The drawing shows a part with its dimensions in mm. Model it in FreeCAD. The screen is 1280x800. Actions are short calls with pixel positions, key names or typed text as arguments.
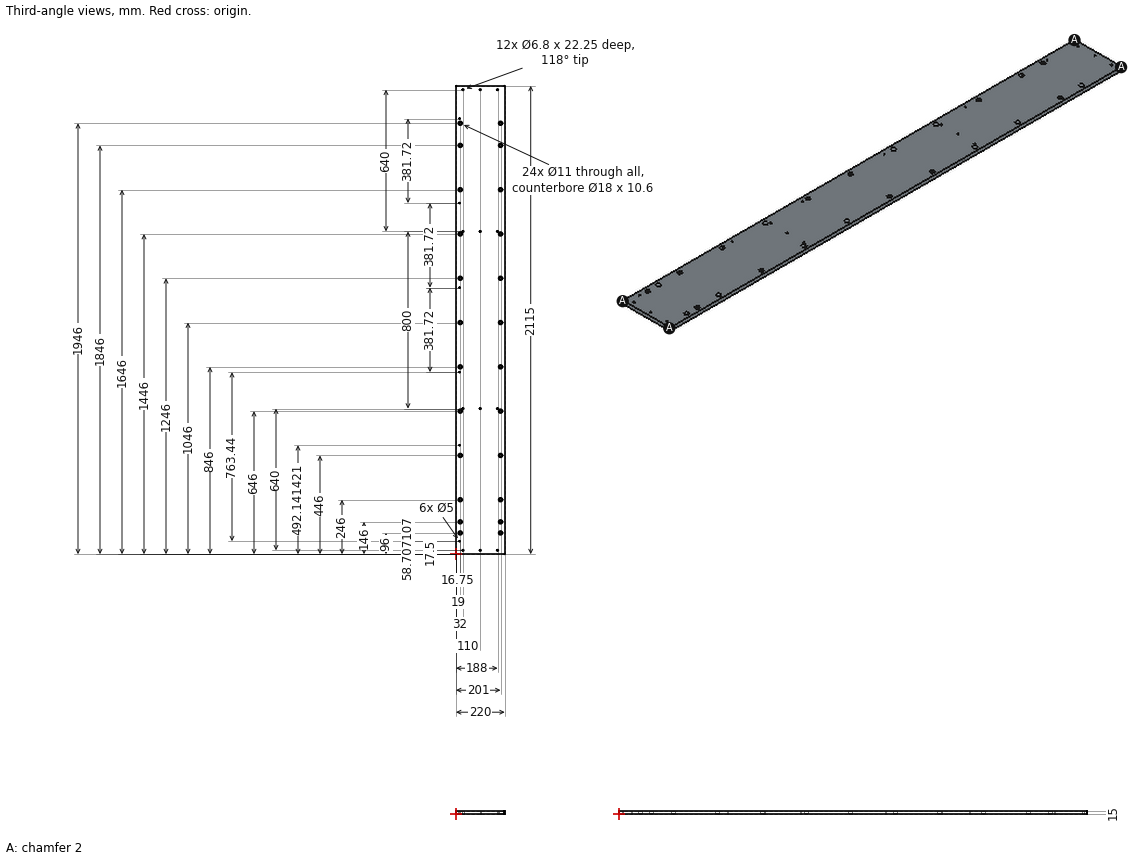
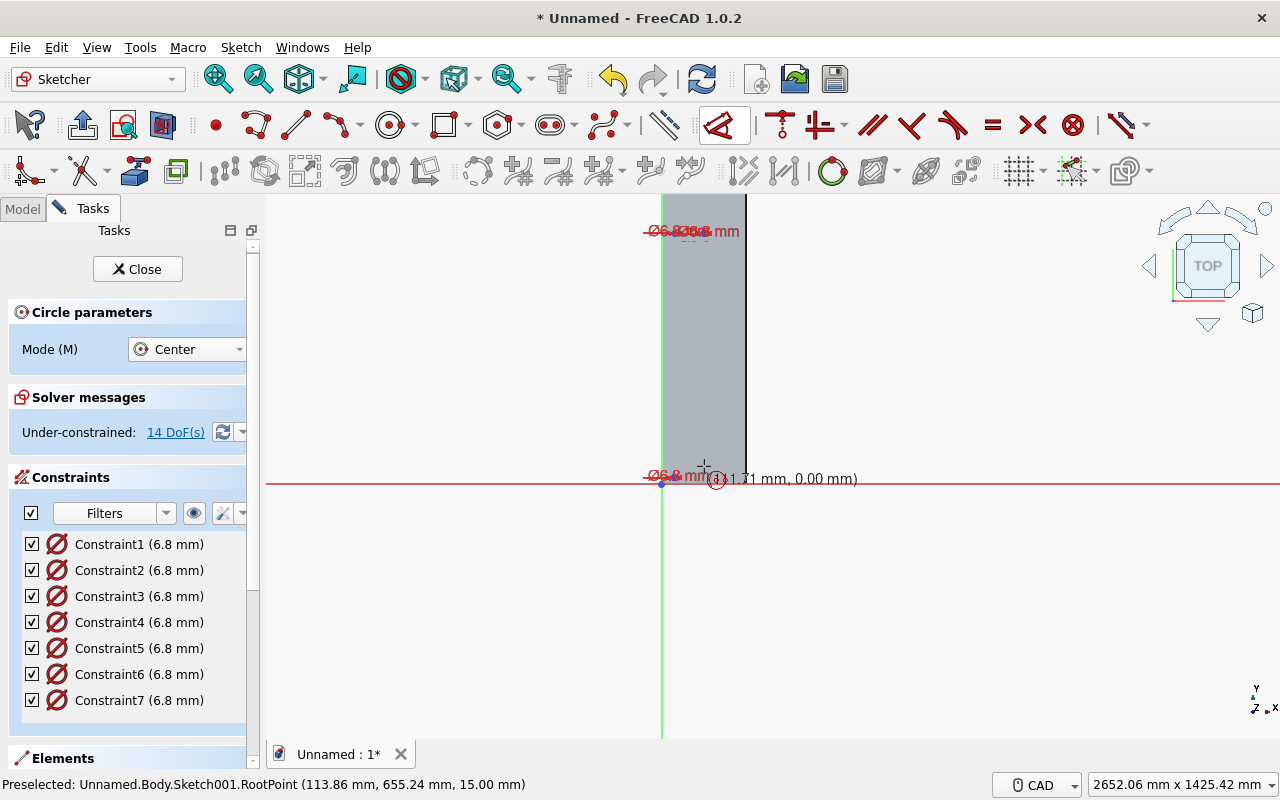
scroll(710, 711, down, 4)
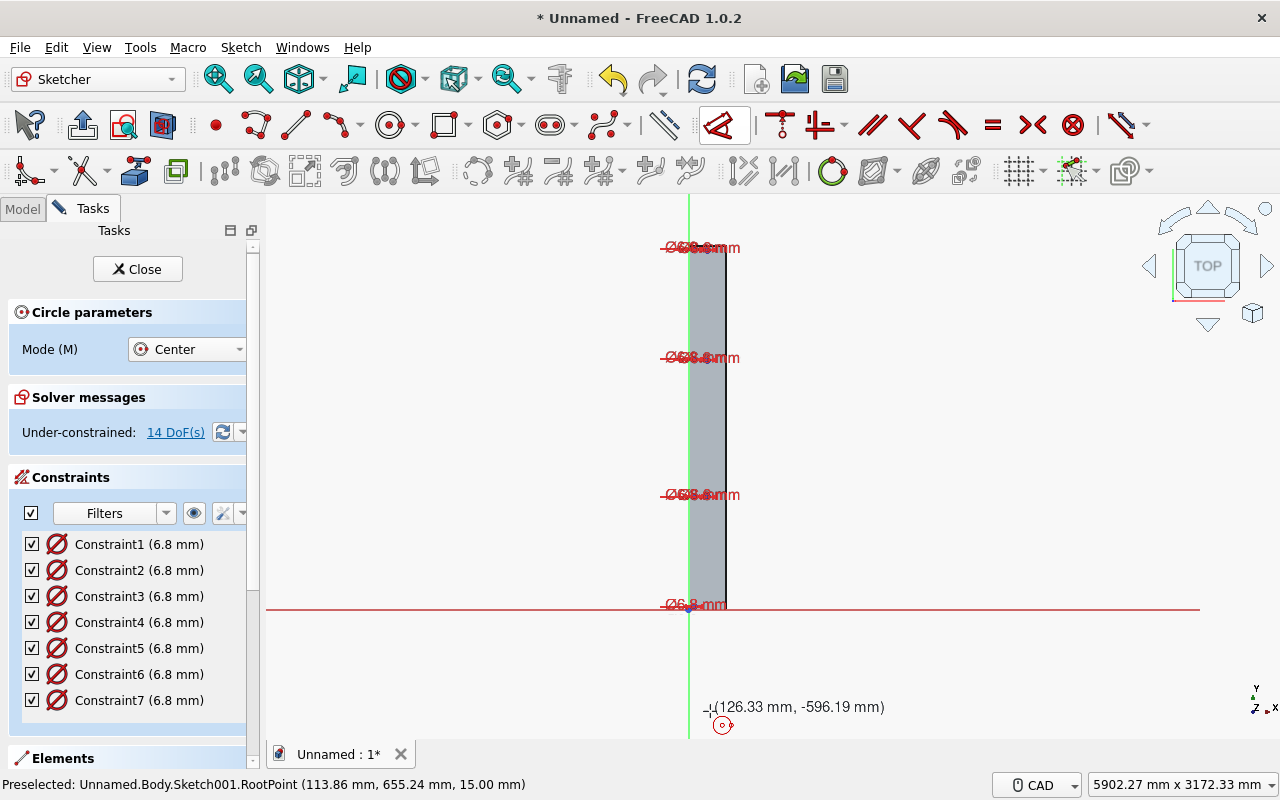
scroll(707, 607, up, 9)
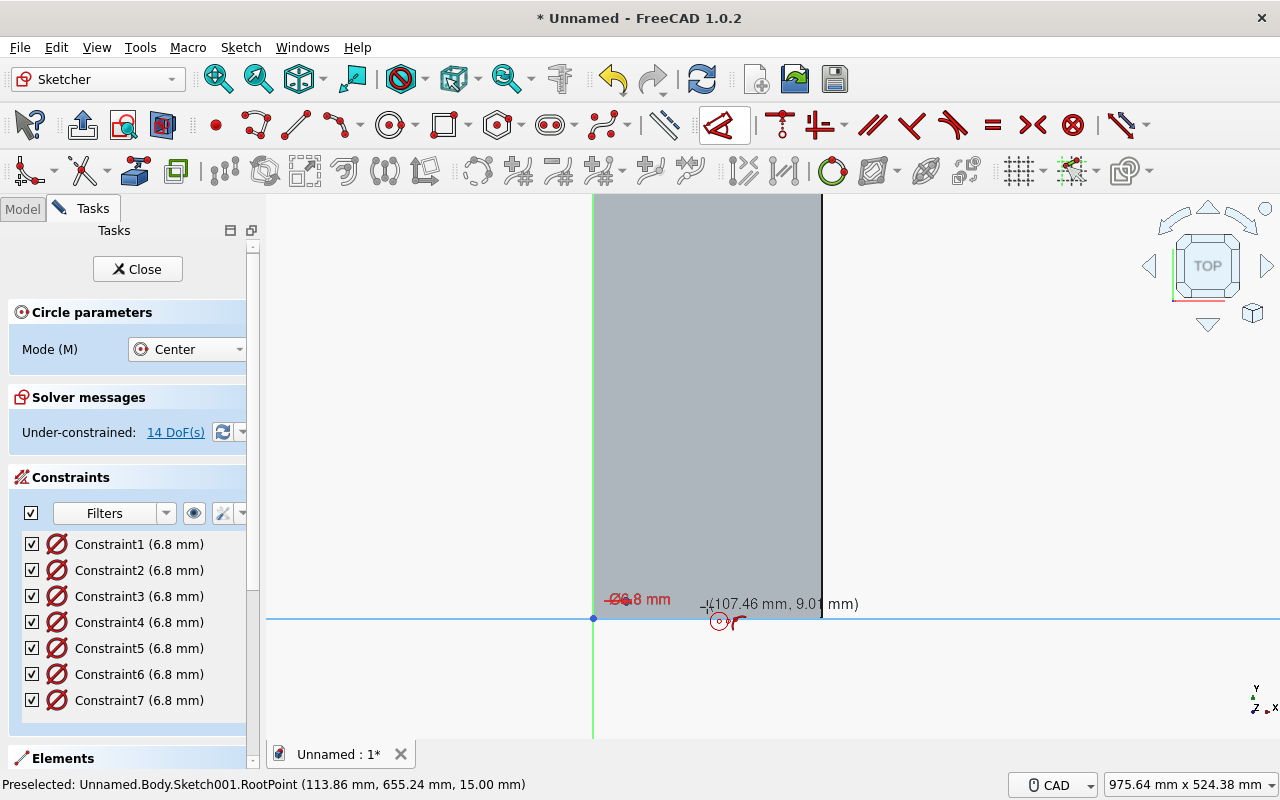
click(707, 600)
move(710, 598)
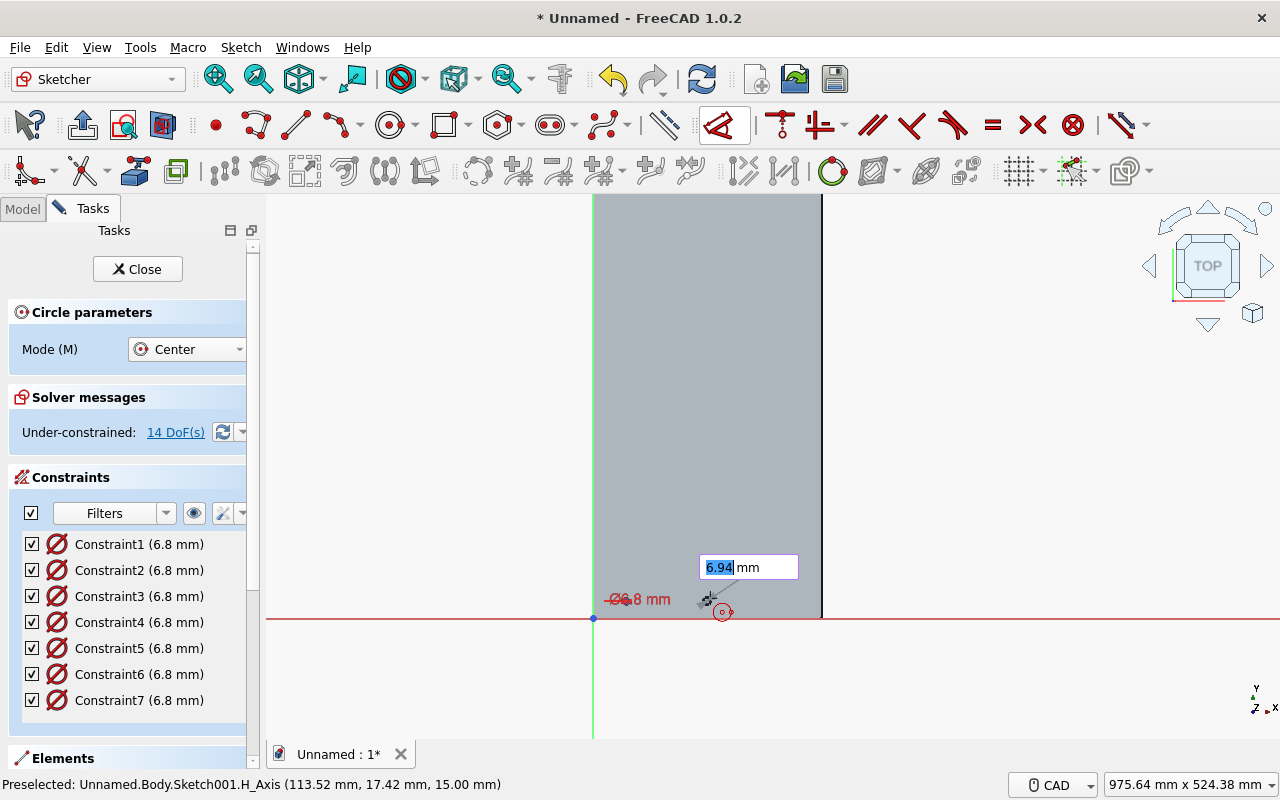
text(6.8)
key(Return)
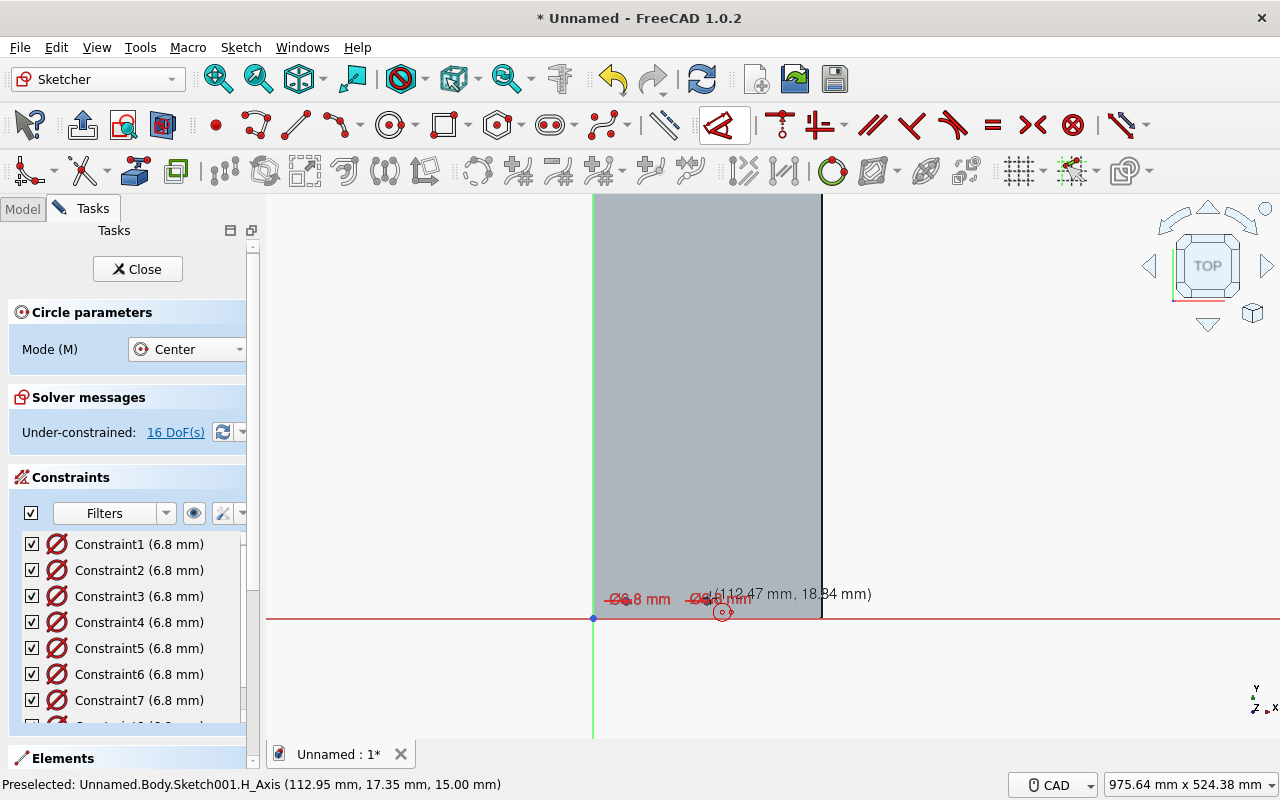
scroll(707, 653, down, 9)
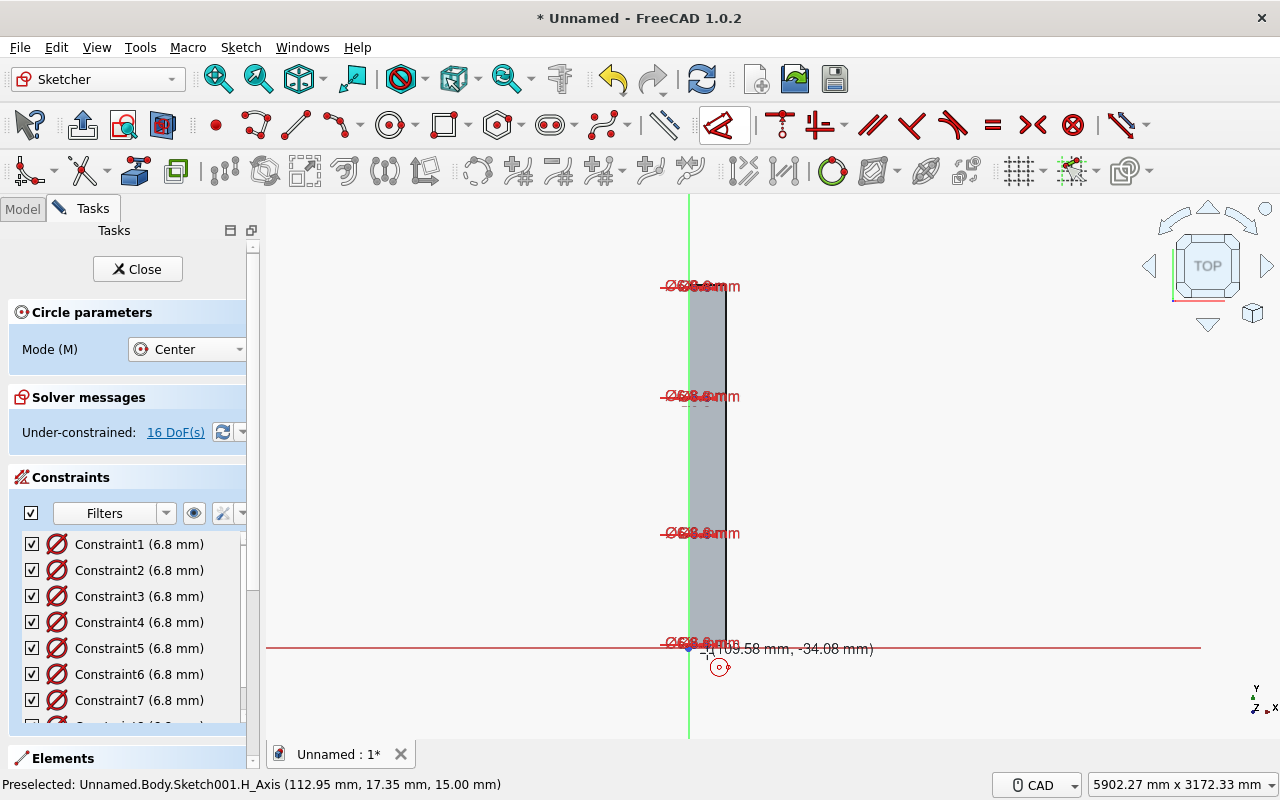
scroll(721, 288, up, 19)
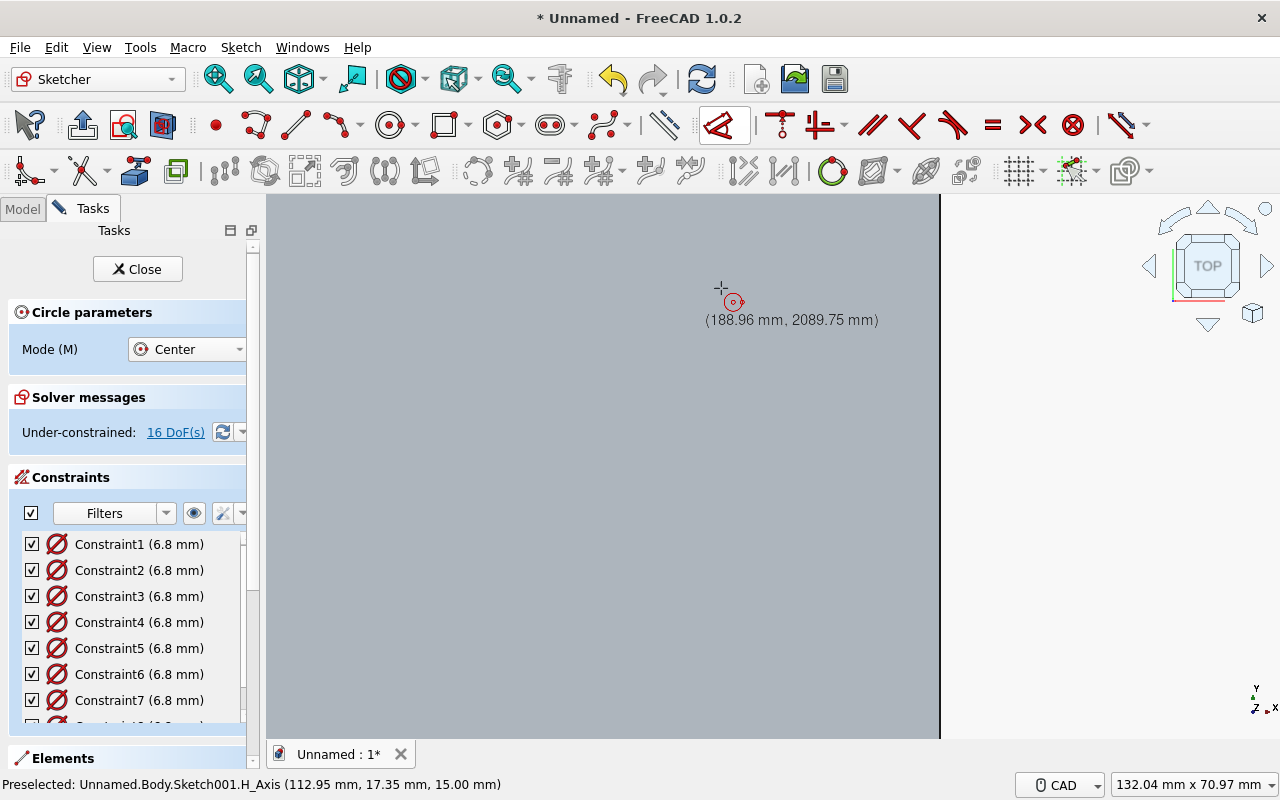
scroll(704, 466, down, 15)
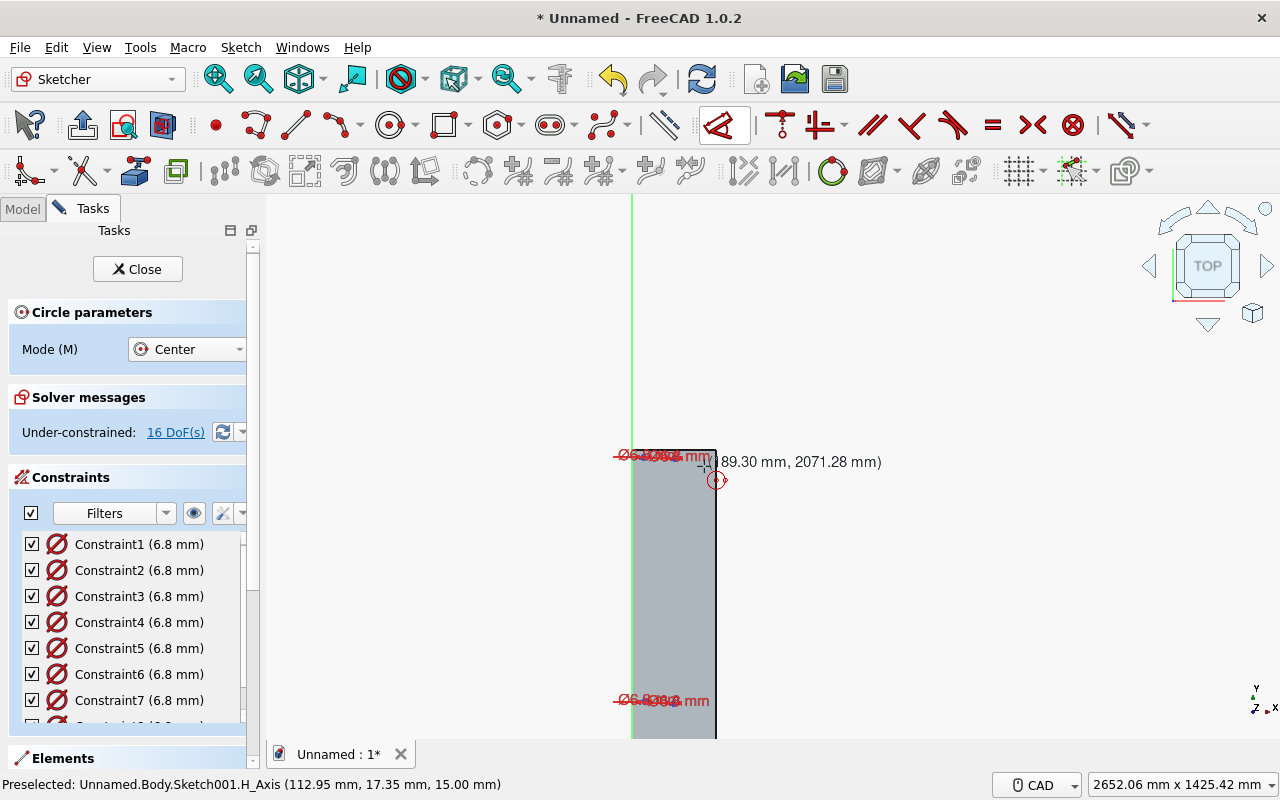
scroll(725, 239, down, 5)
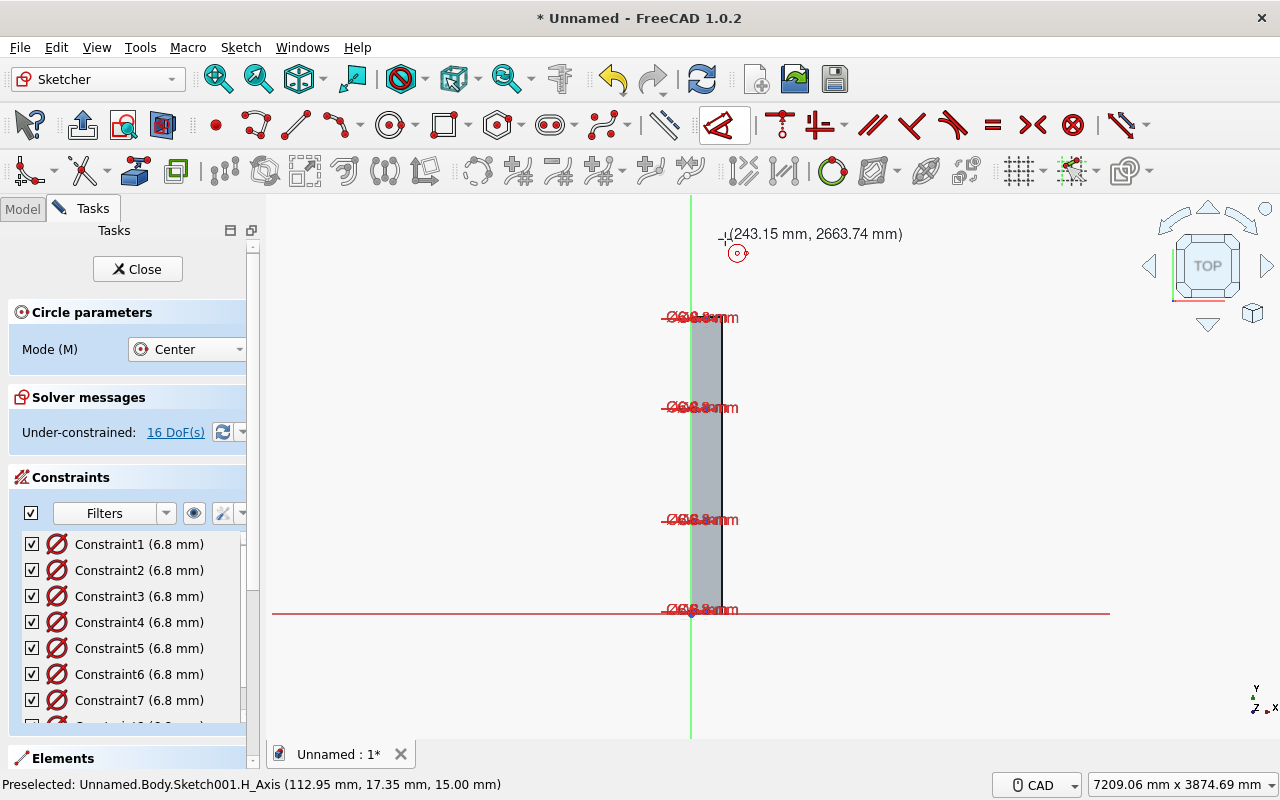
scroll(718, 319, up, 3)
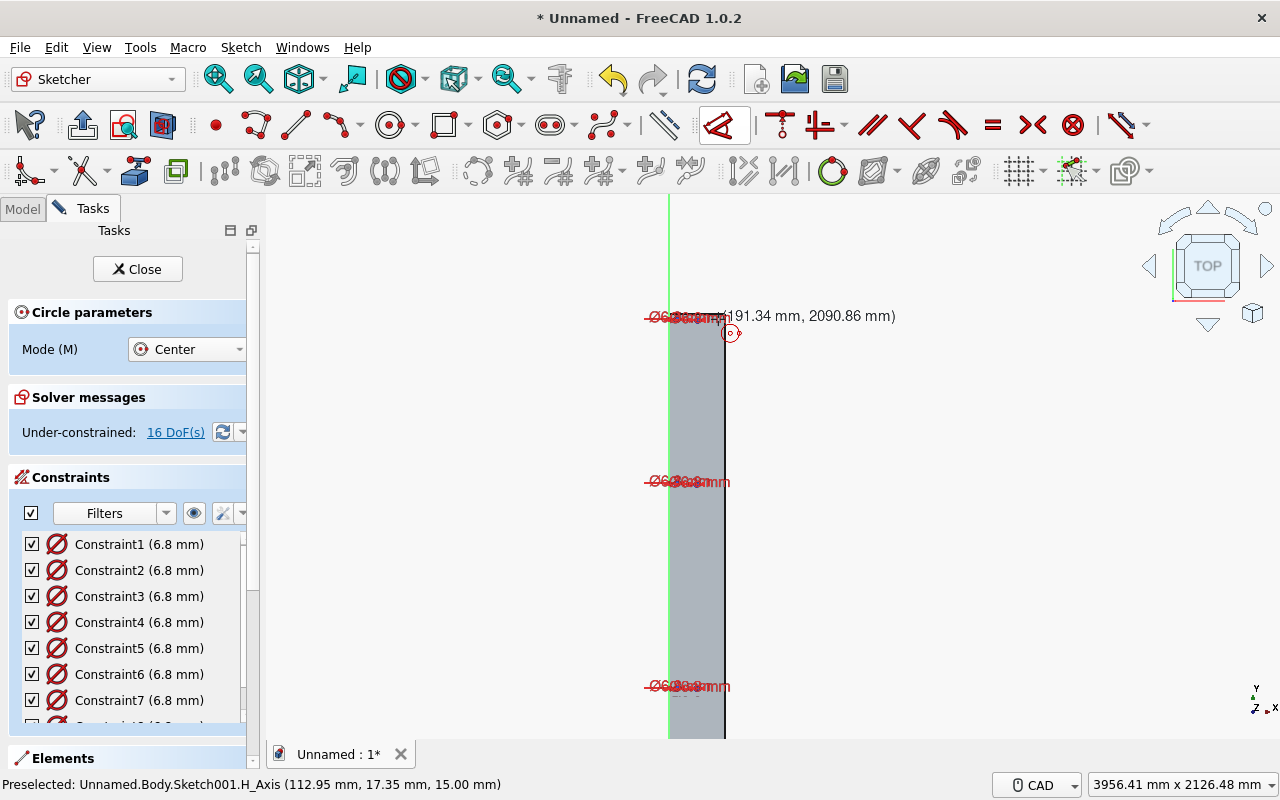
click(717, 319)
move(717, 318)